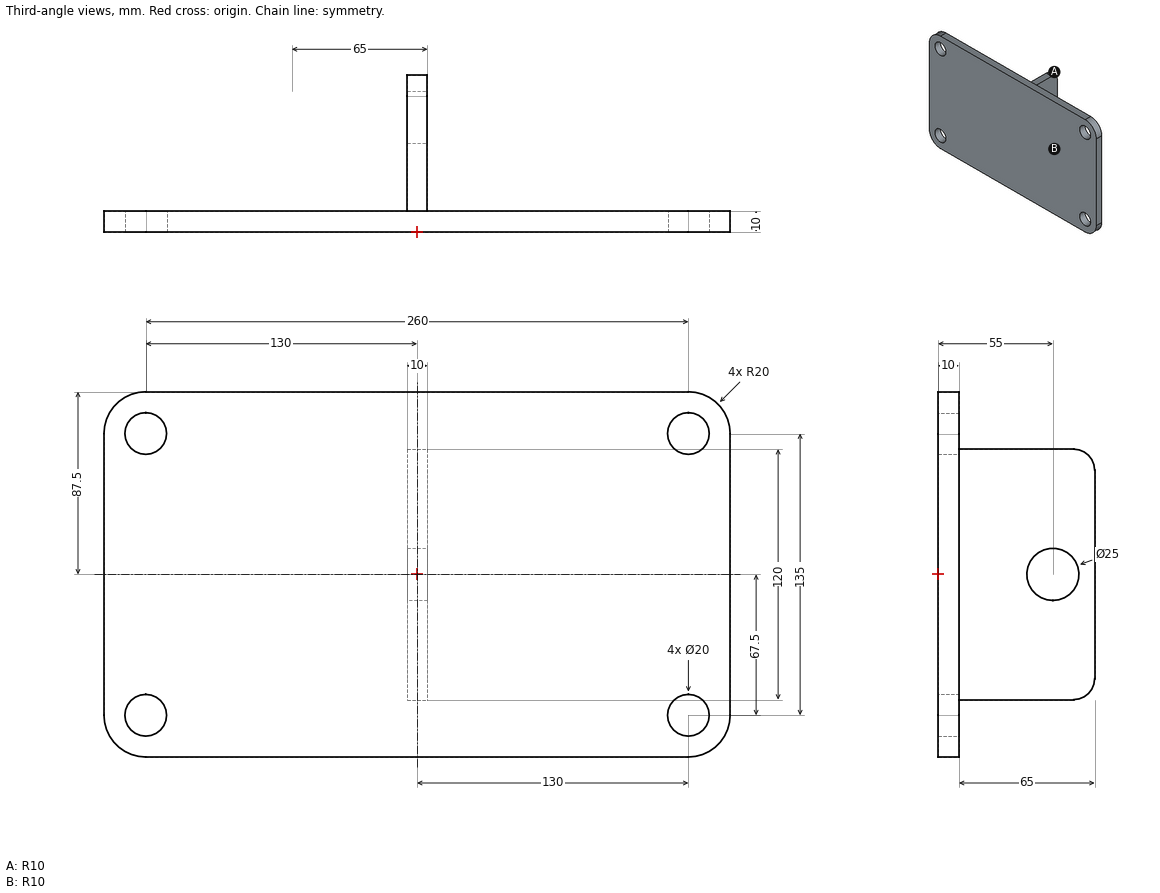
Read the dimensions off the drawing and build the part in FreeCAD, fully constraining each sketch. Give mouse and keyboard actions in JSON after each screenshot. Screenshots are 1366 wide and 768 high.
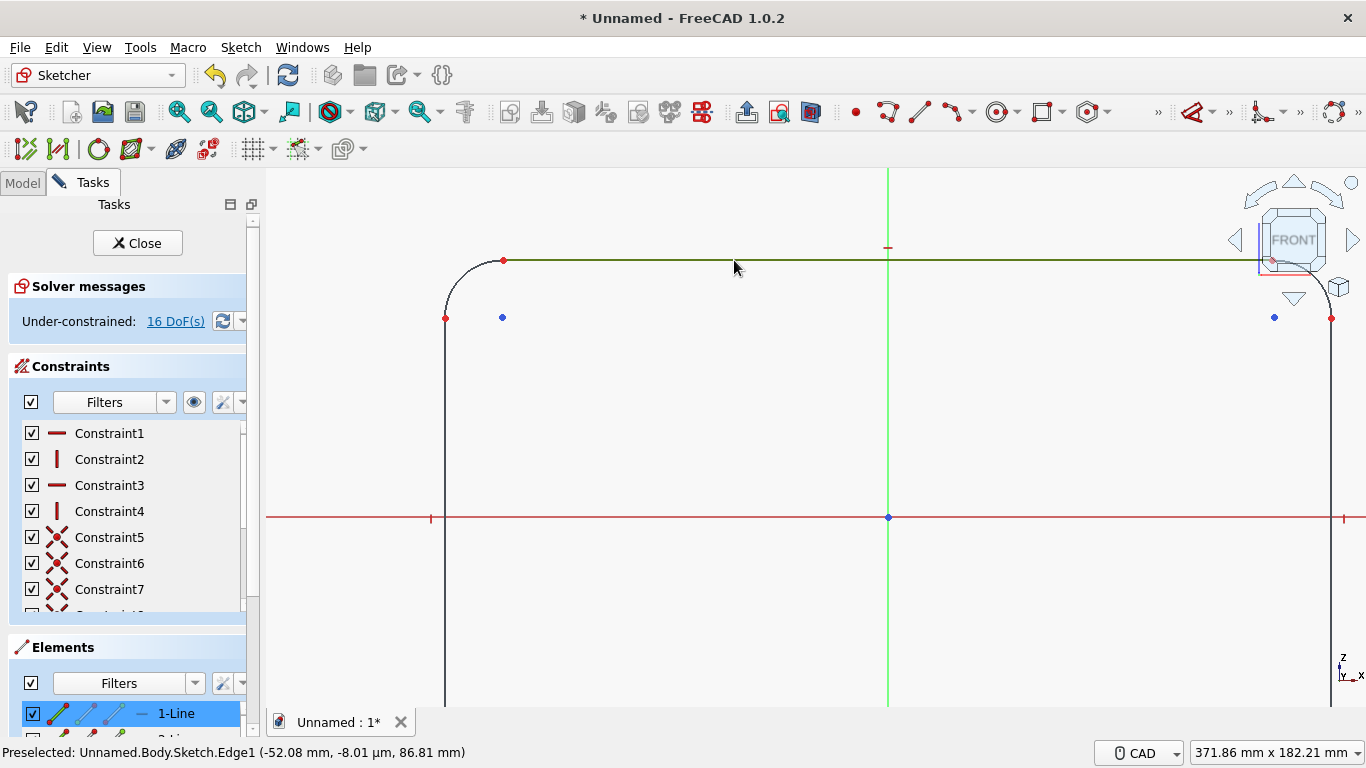
{"action": "scroll", "coordinate": [462, 275], "scroll_direction": "down", "scroll_amount": 2}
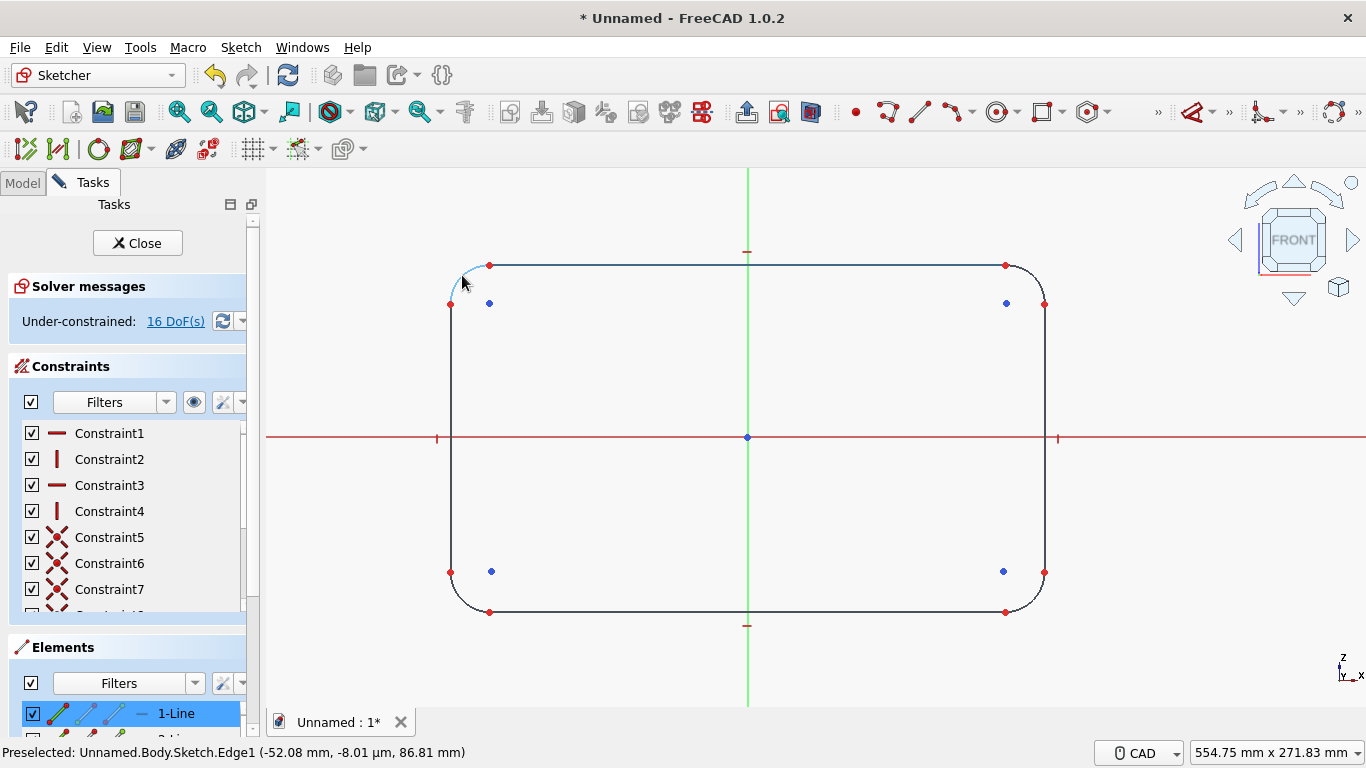
{"action": "left_click", "coordinate": [1041, 286]}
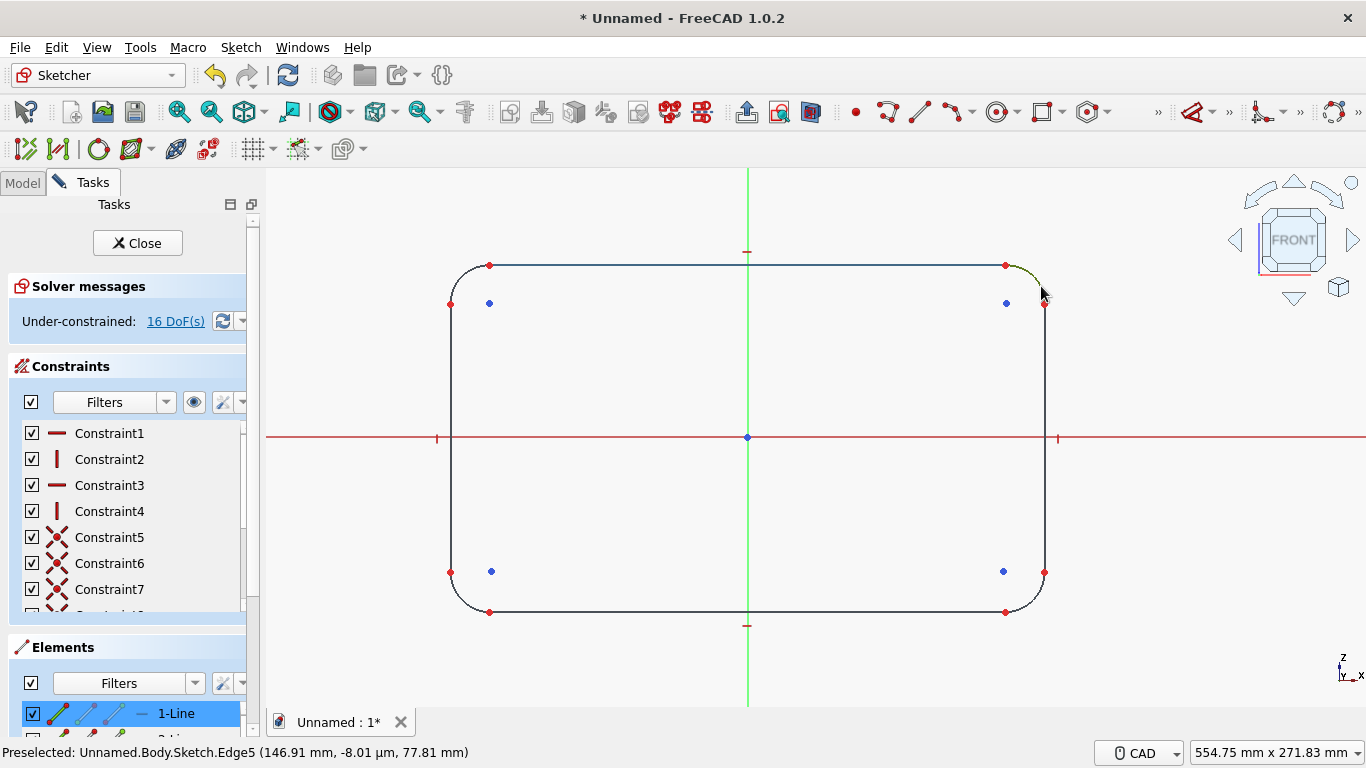
{"action": "key", "text": "t"}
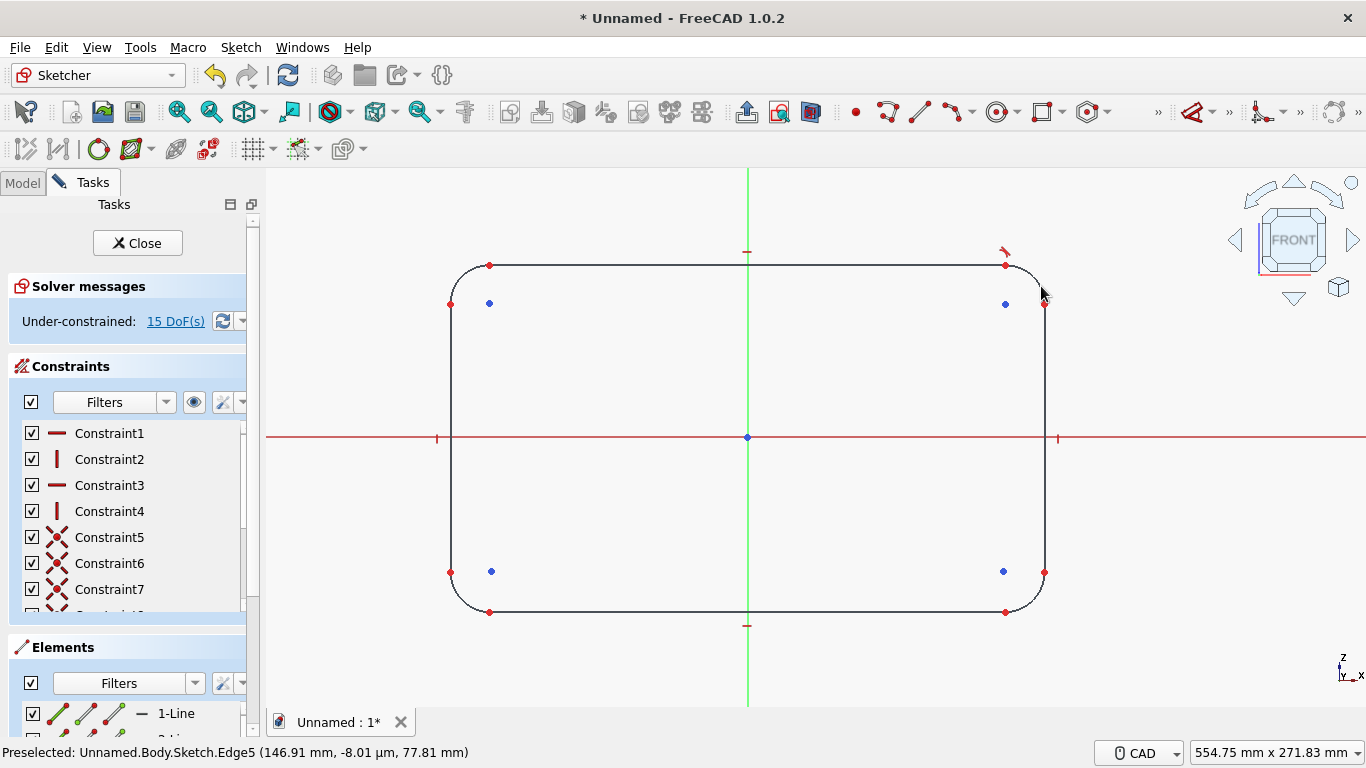
{"action": "left_click", "coordinate": [644, 265]}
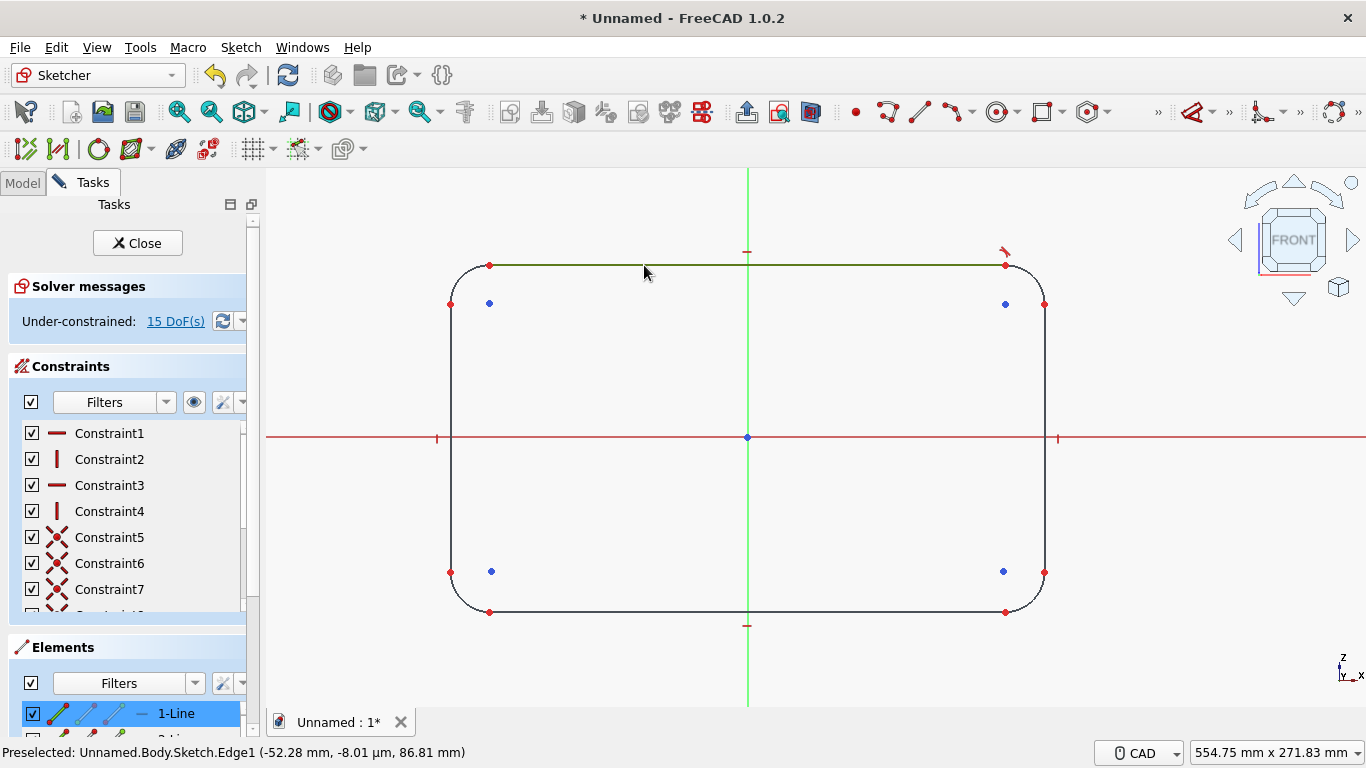
{"action": "left_click", "coordinate": [472, 269]}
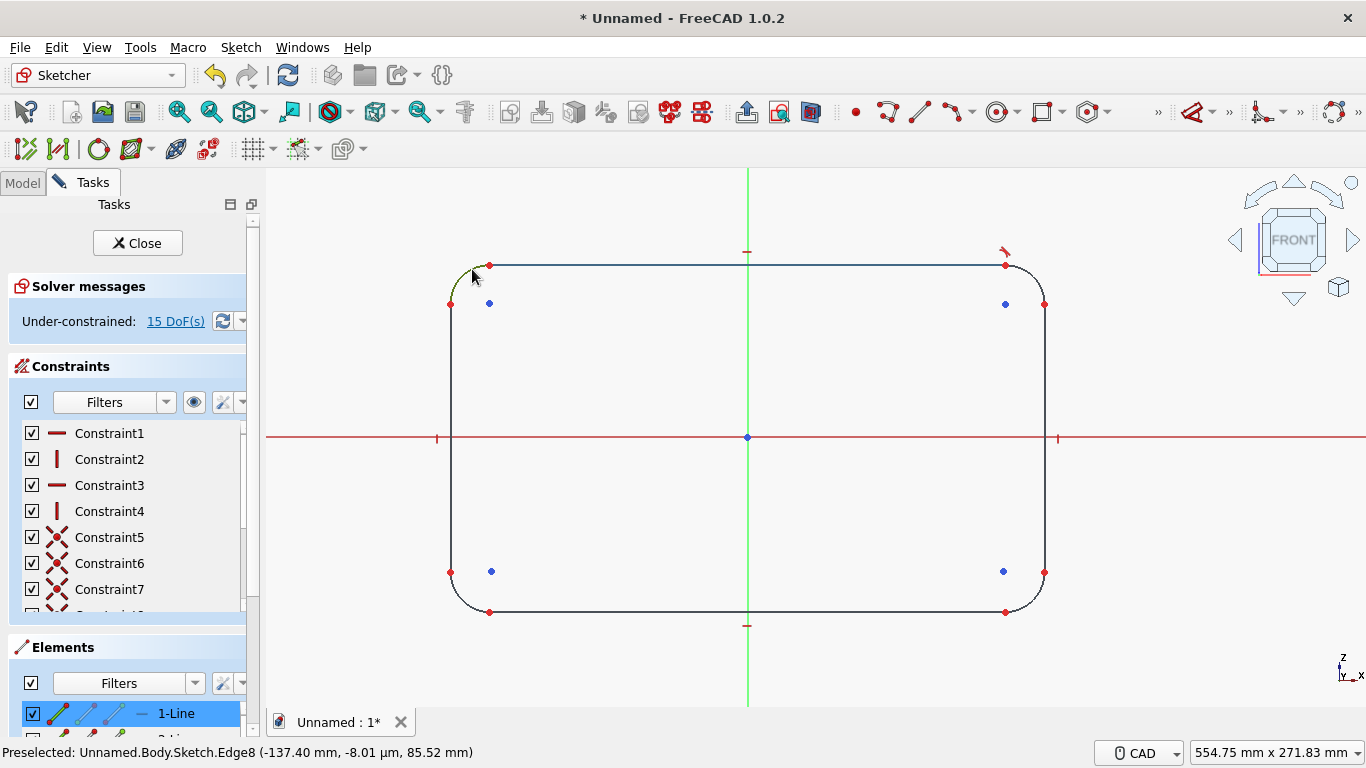
{"action": "key", "text": "t"}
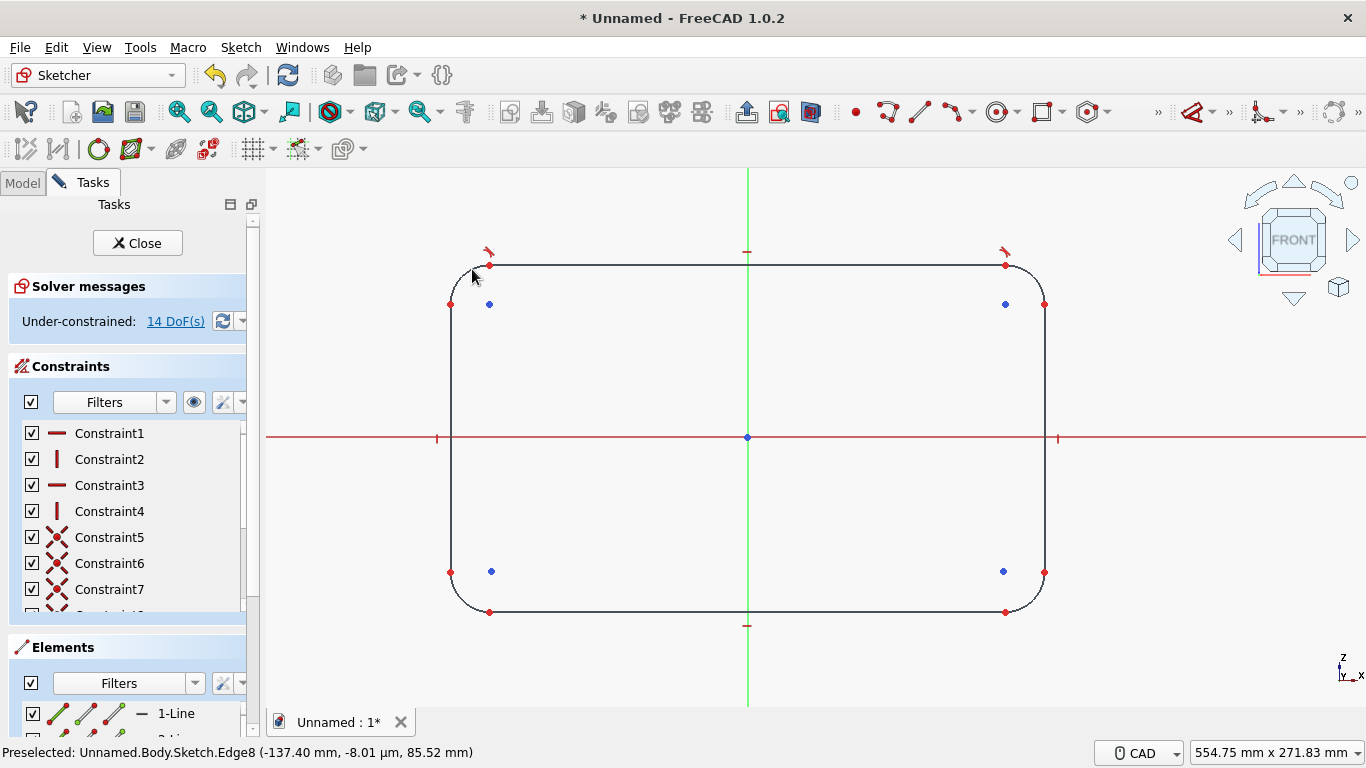
{"action": "left_click", "coordinate": [1045, 385]}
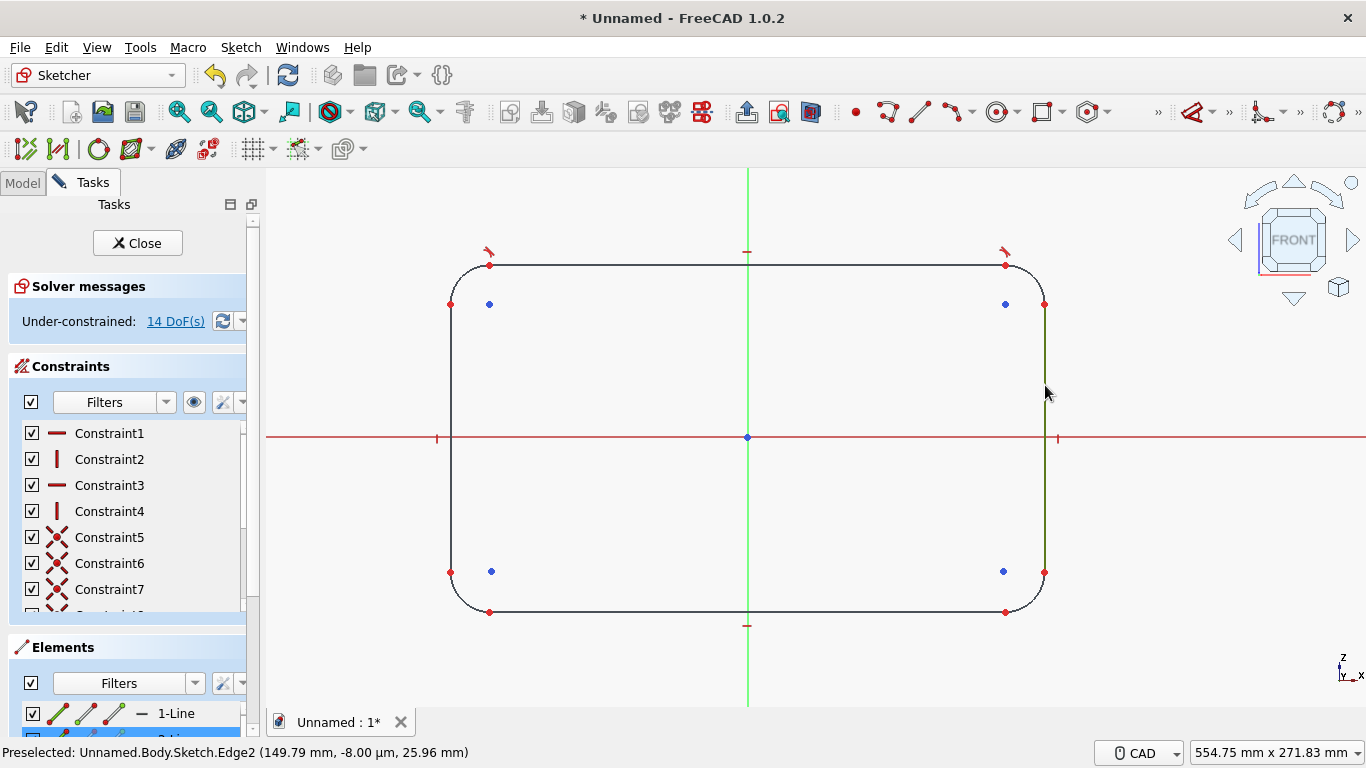
{"action": "left_click", "coordinate": [1040, 287]}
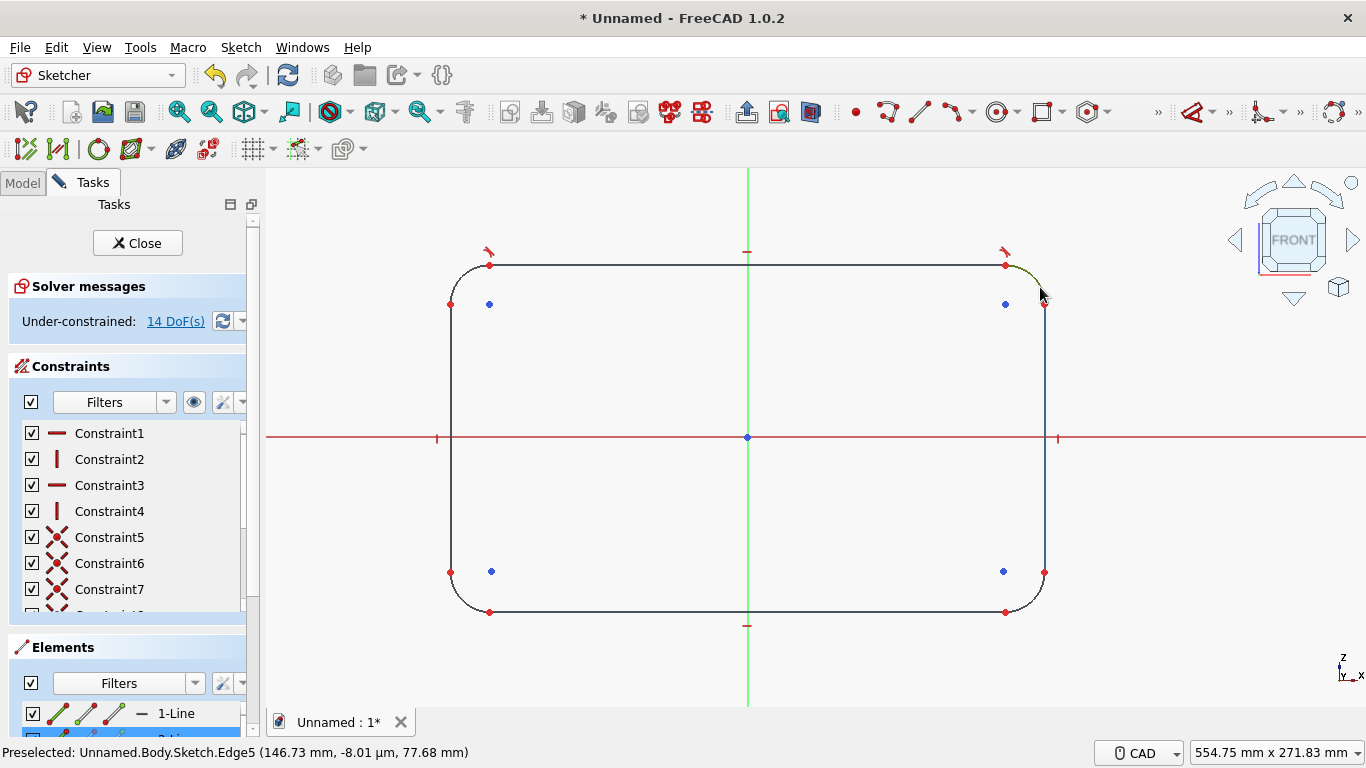
{"action": "key", "text": "t"}